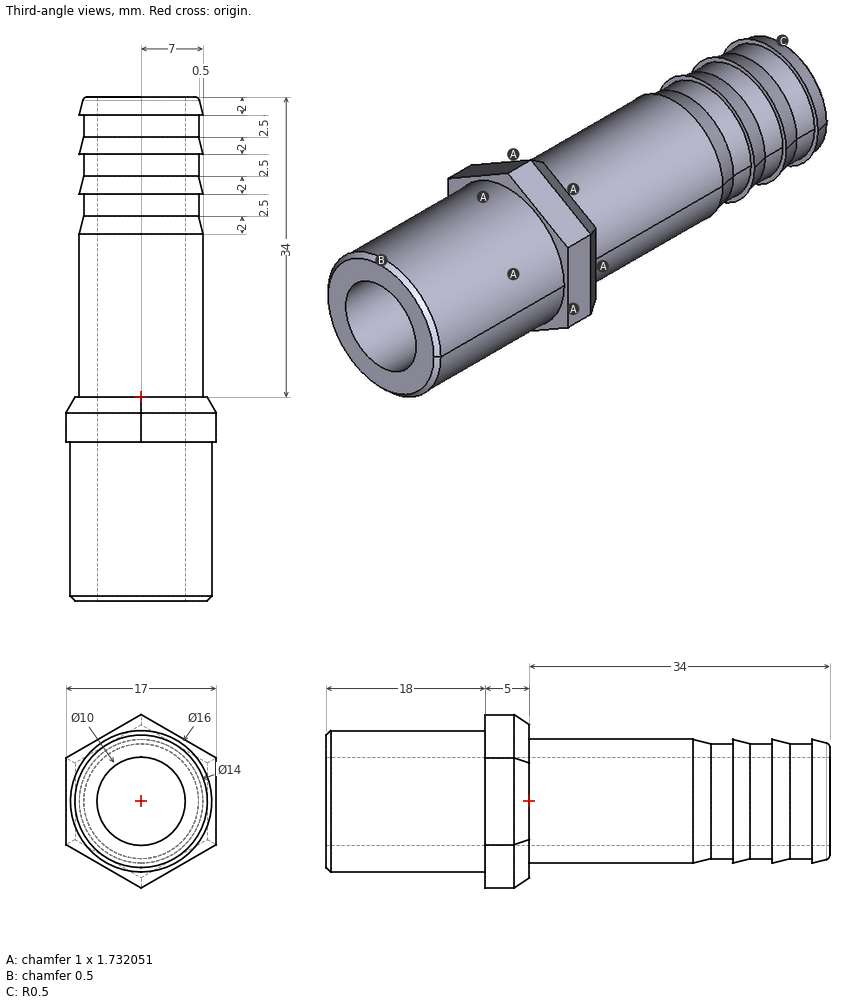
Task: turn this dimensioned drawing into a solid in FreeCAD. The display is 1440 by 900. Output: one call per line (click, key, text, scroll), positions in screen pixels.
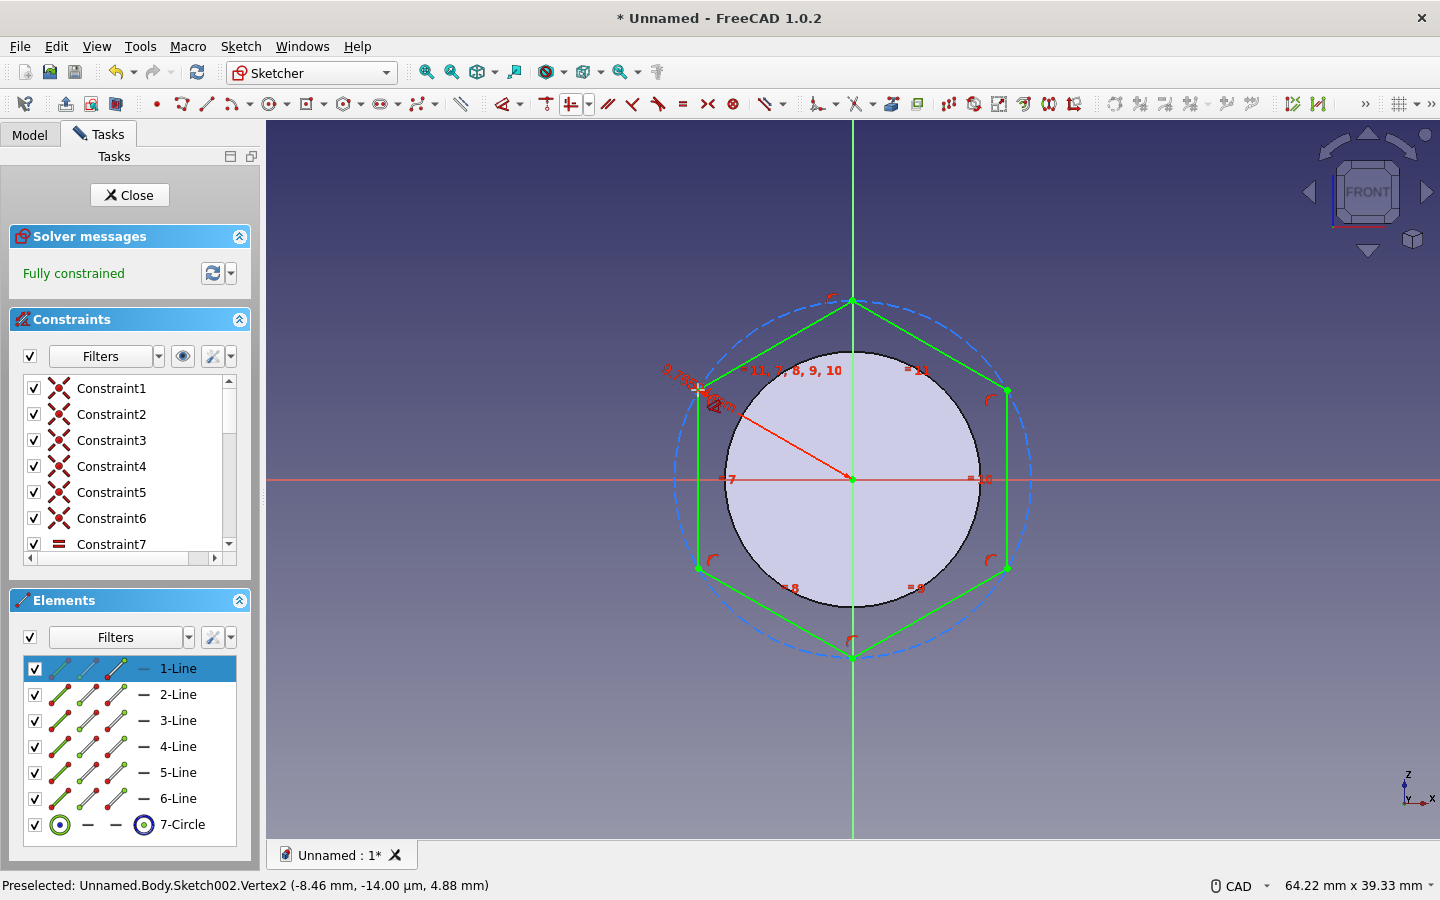
click(1007, 569)
click(745, 651)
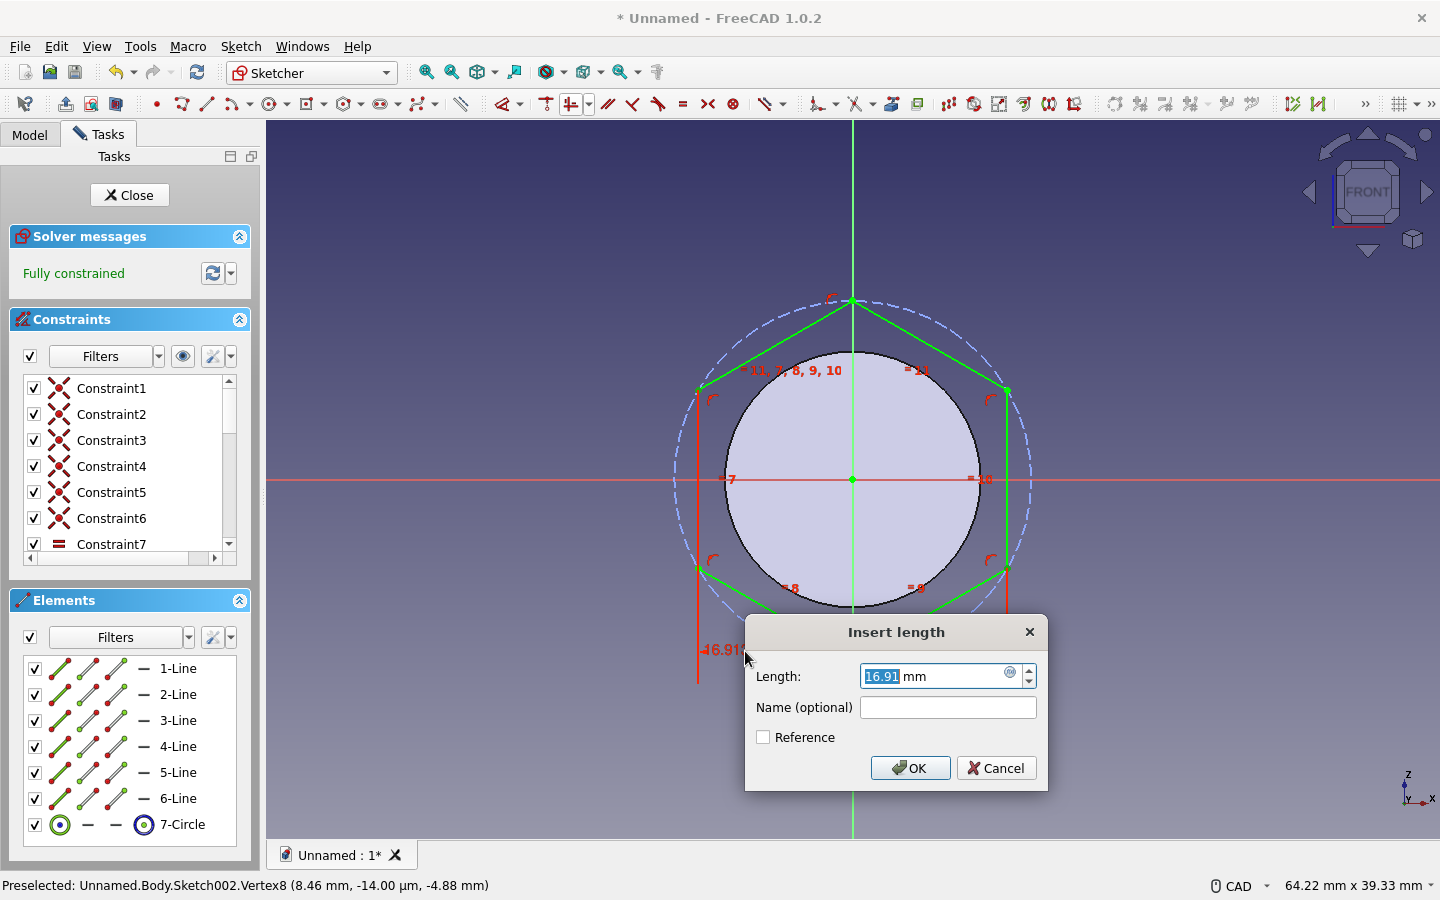
text(17)
key(Return)
key(Escape)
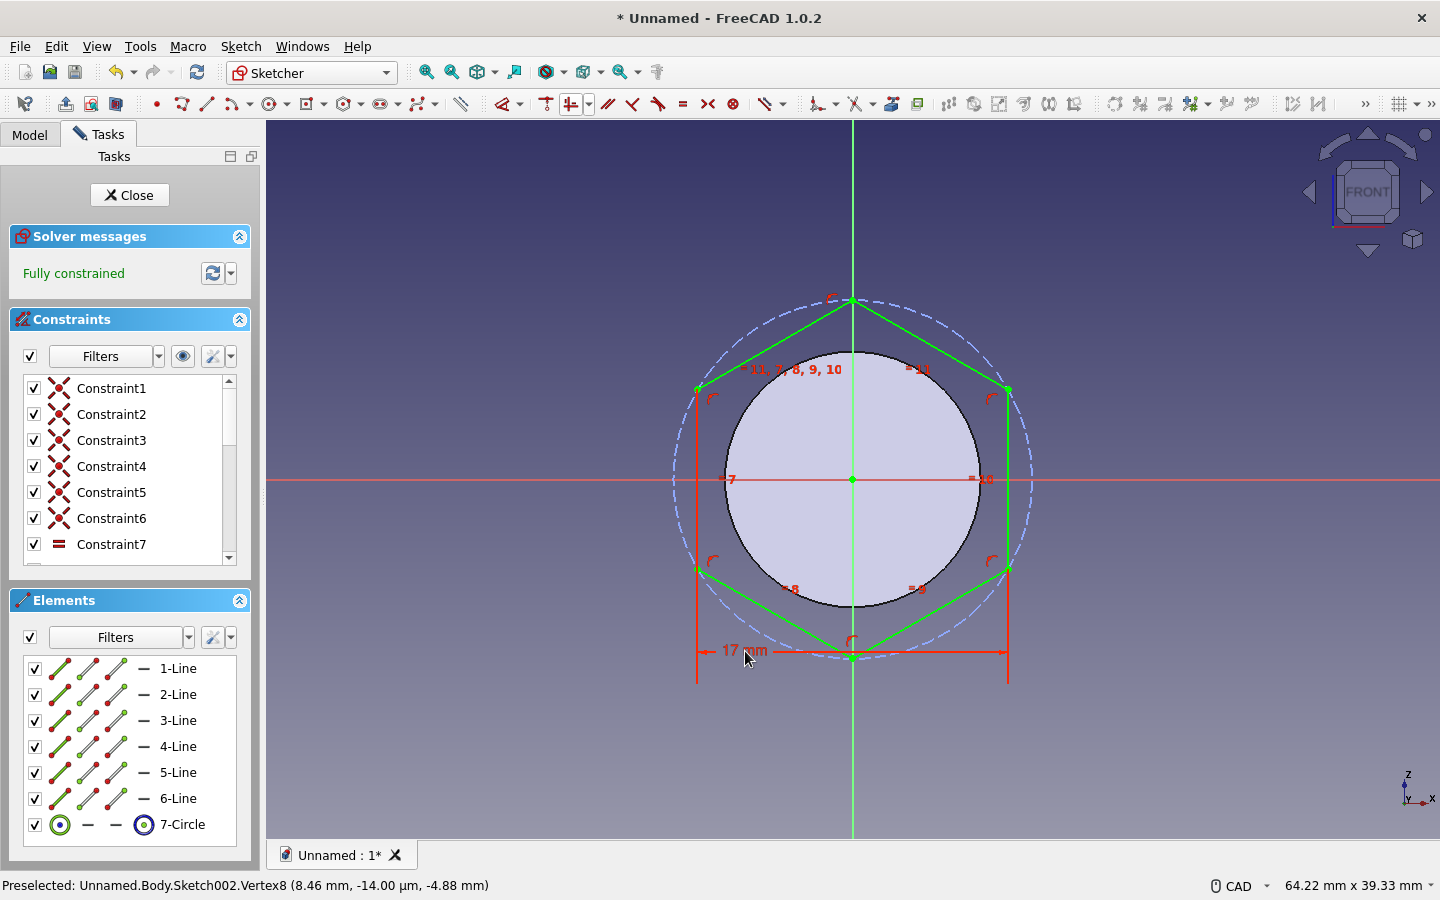
click(130, 195)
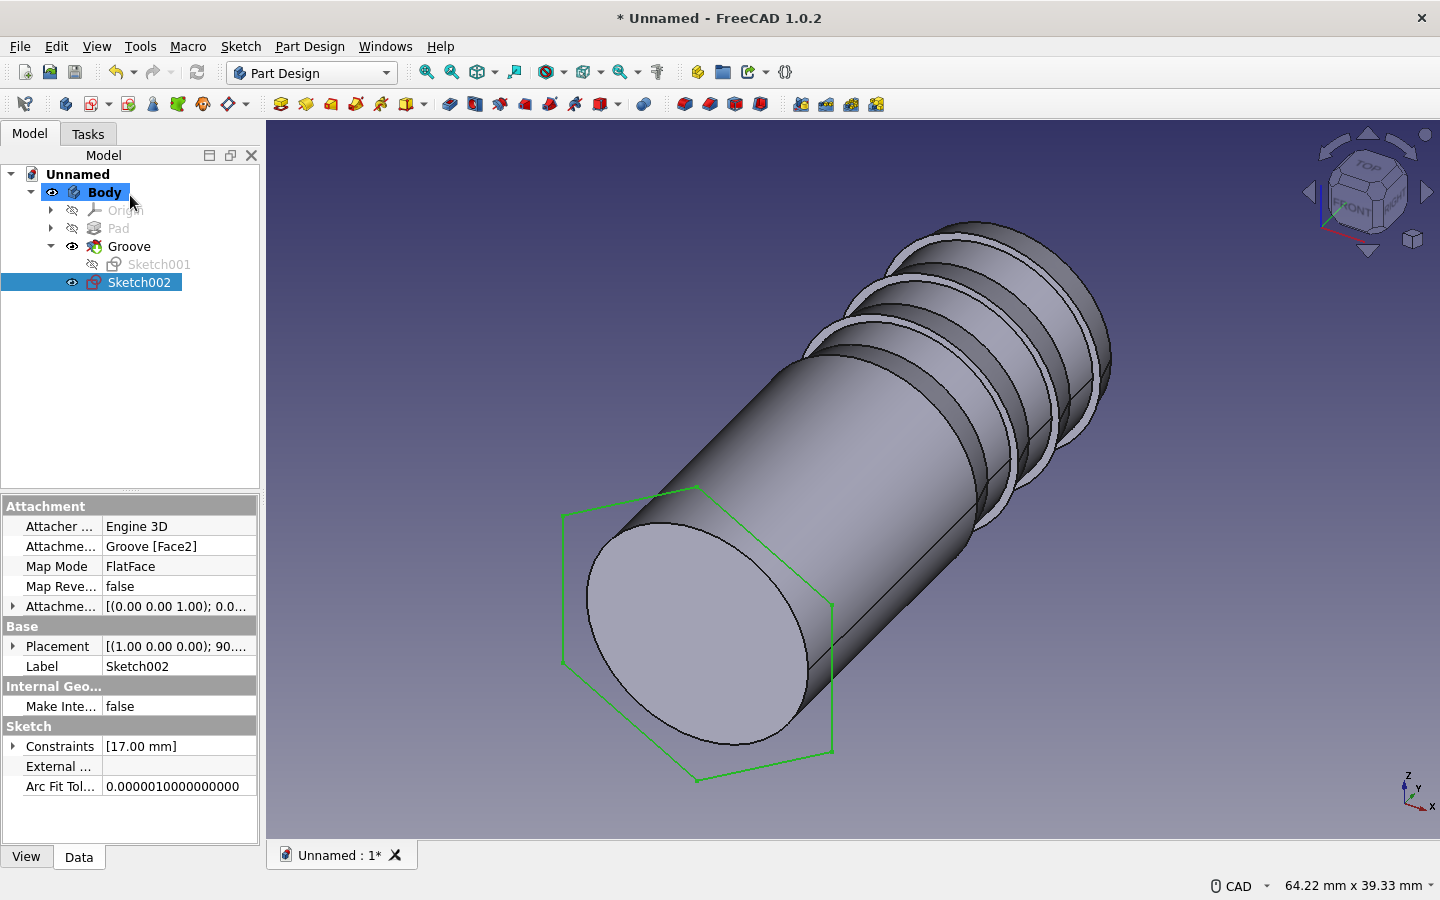
click(281, 104)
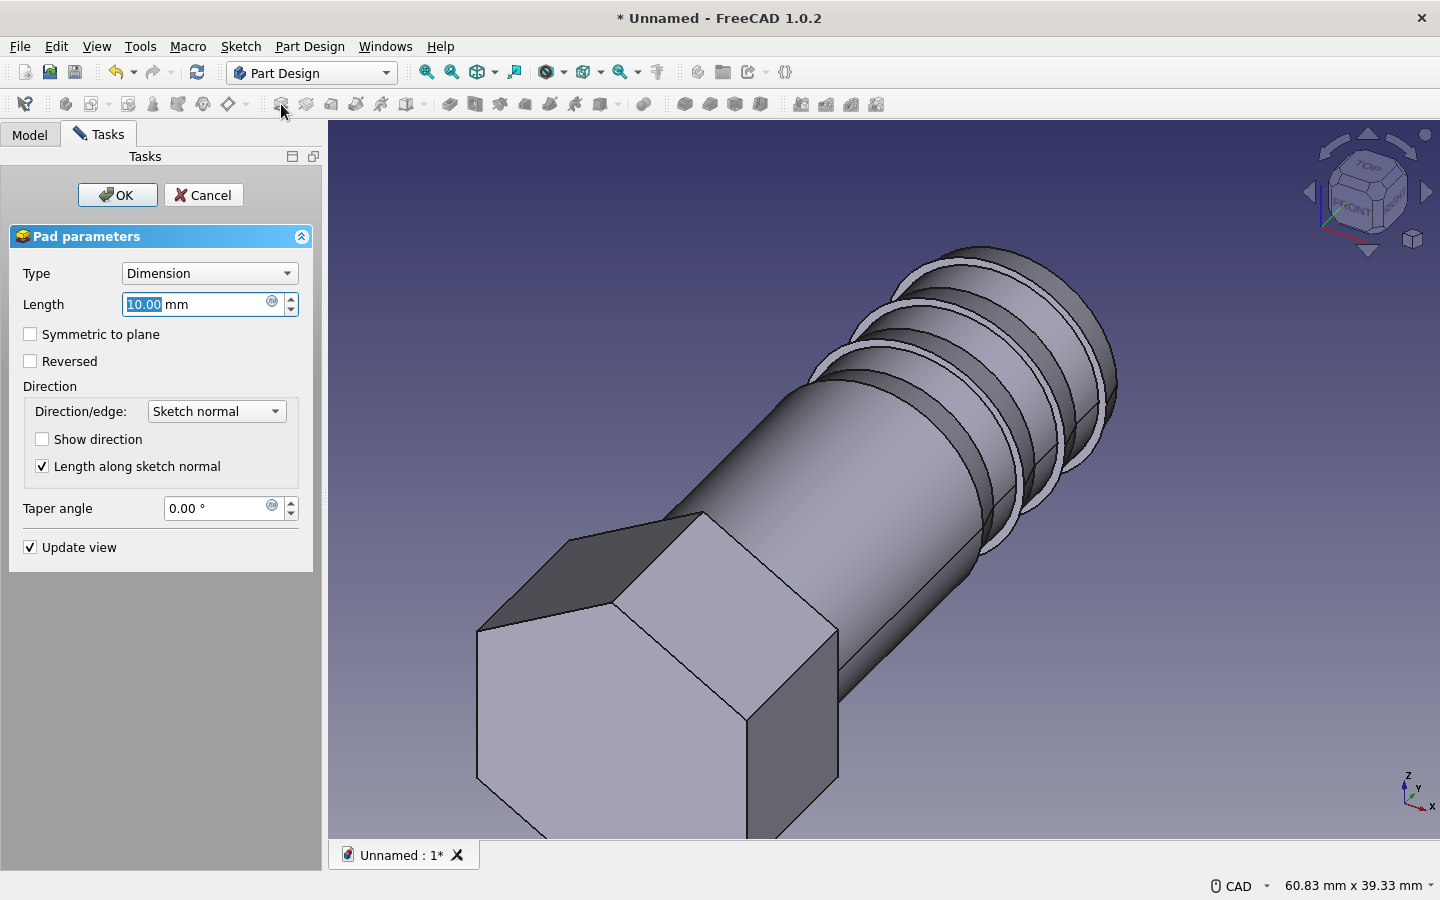
text(5)
key(Tab)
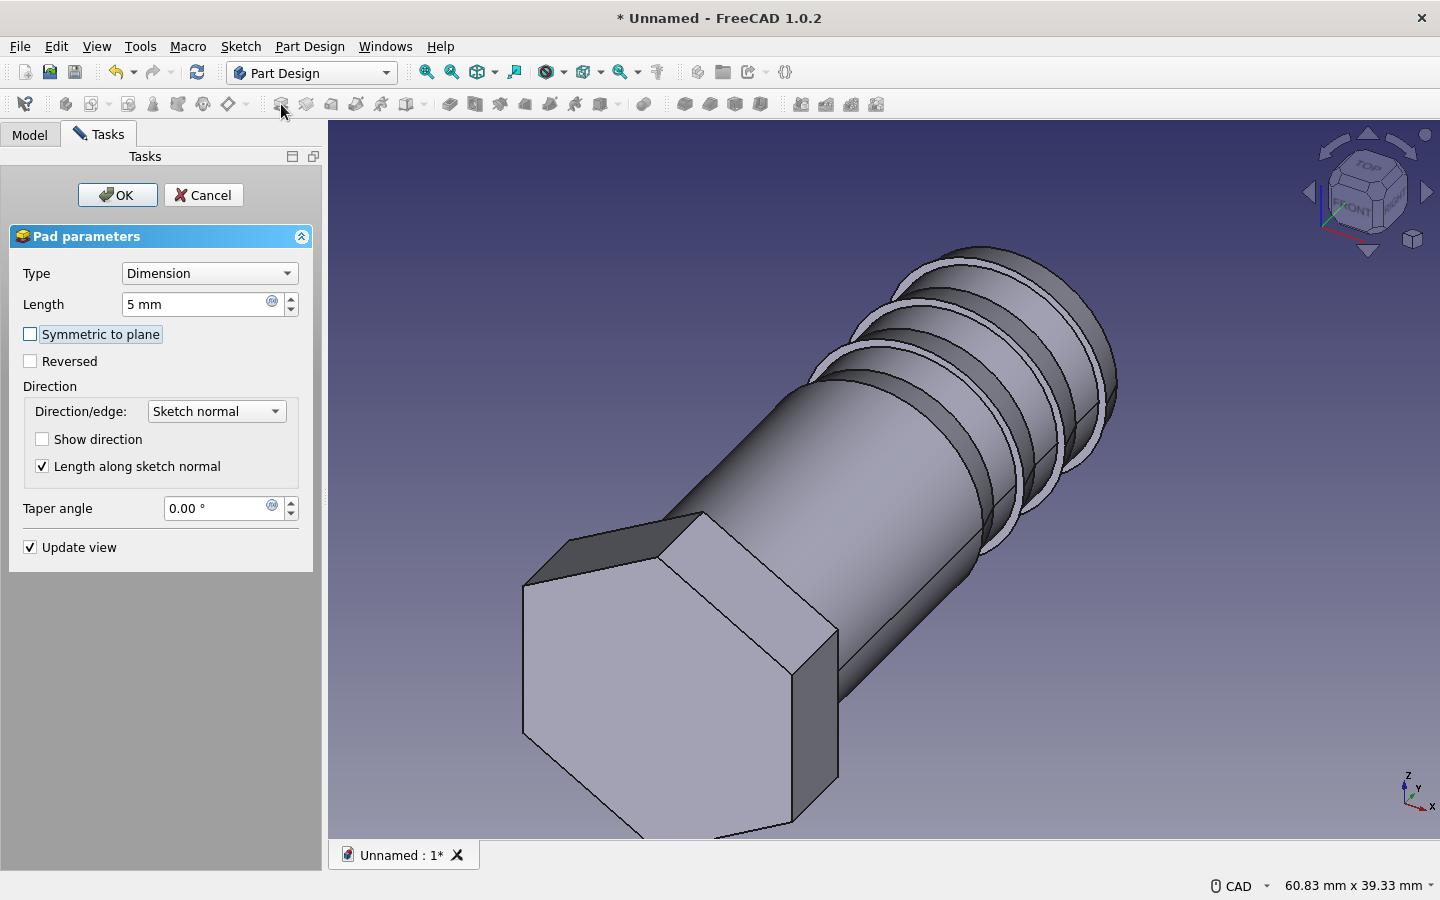
click(118, 195)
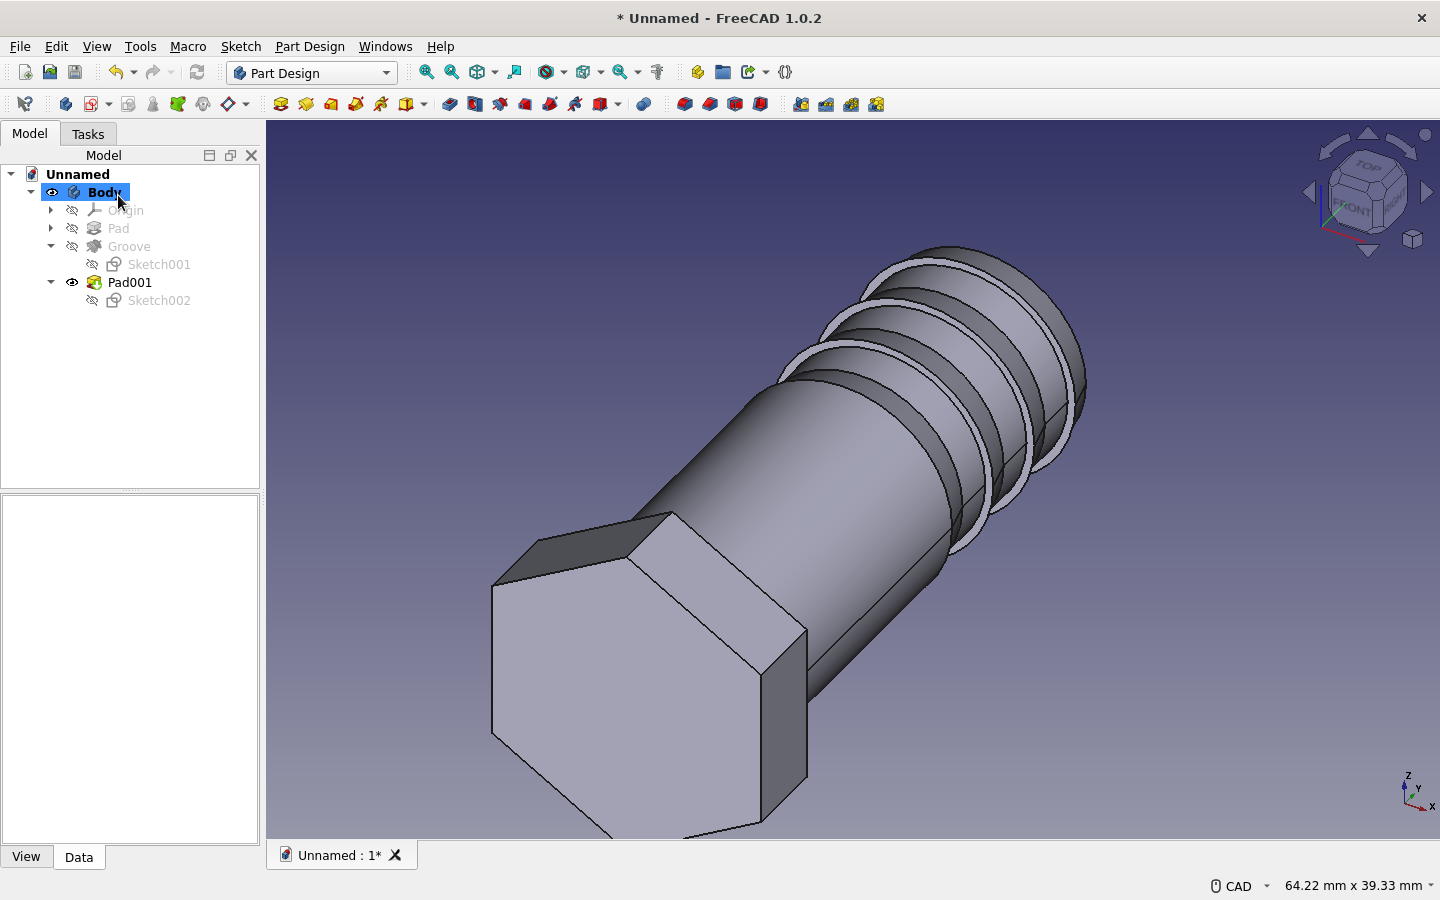
key(v)
key(f)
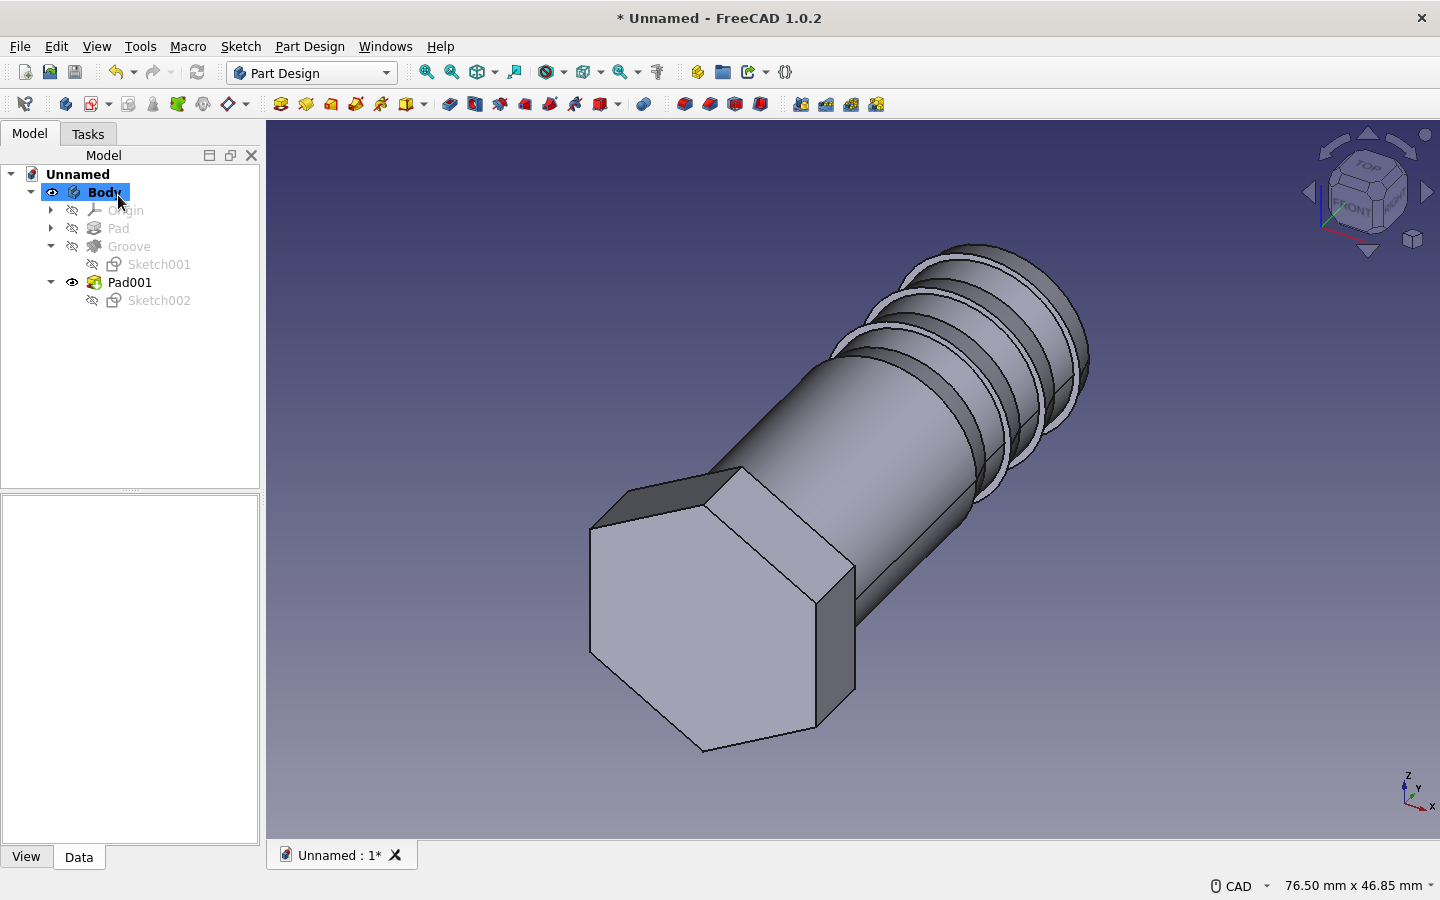
click(703, 627)